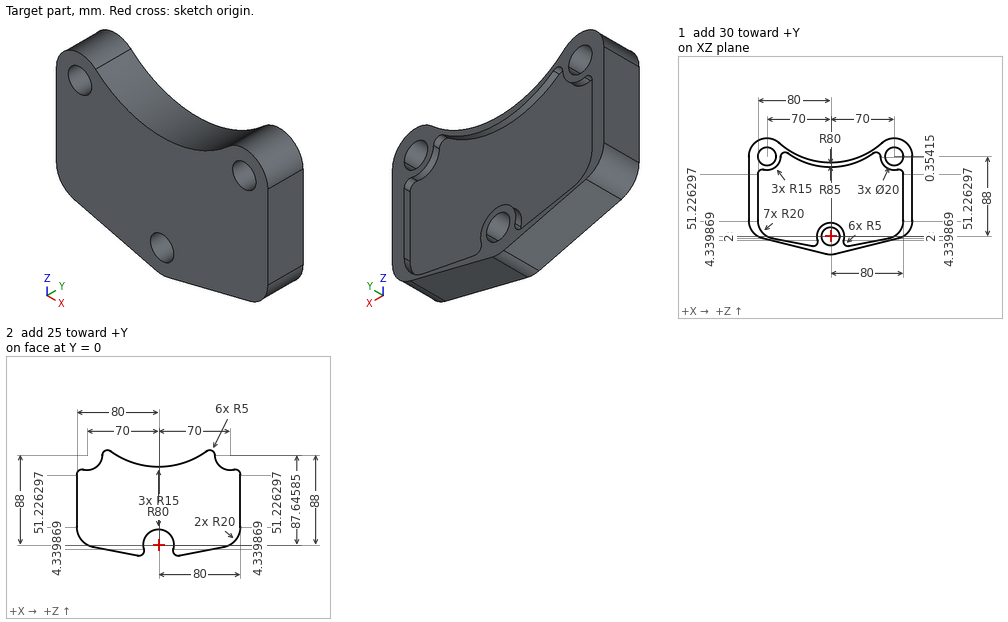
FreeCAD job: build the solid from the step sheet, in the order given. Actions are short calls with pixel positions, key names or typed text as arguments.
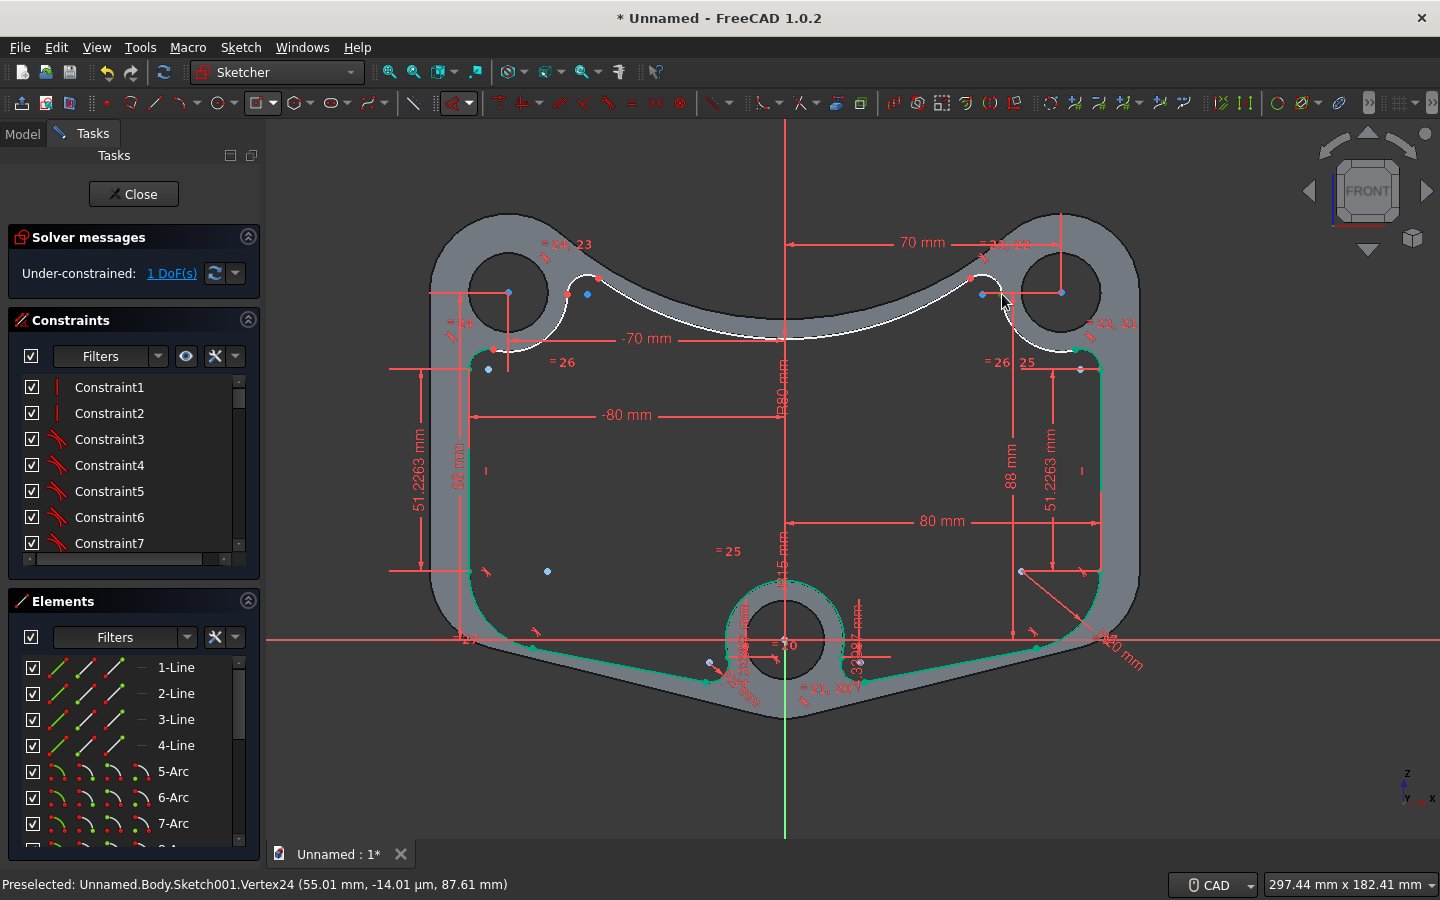
key(i)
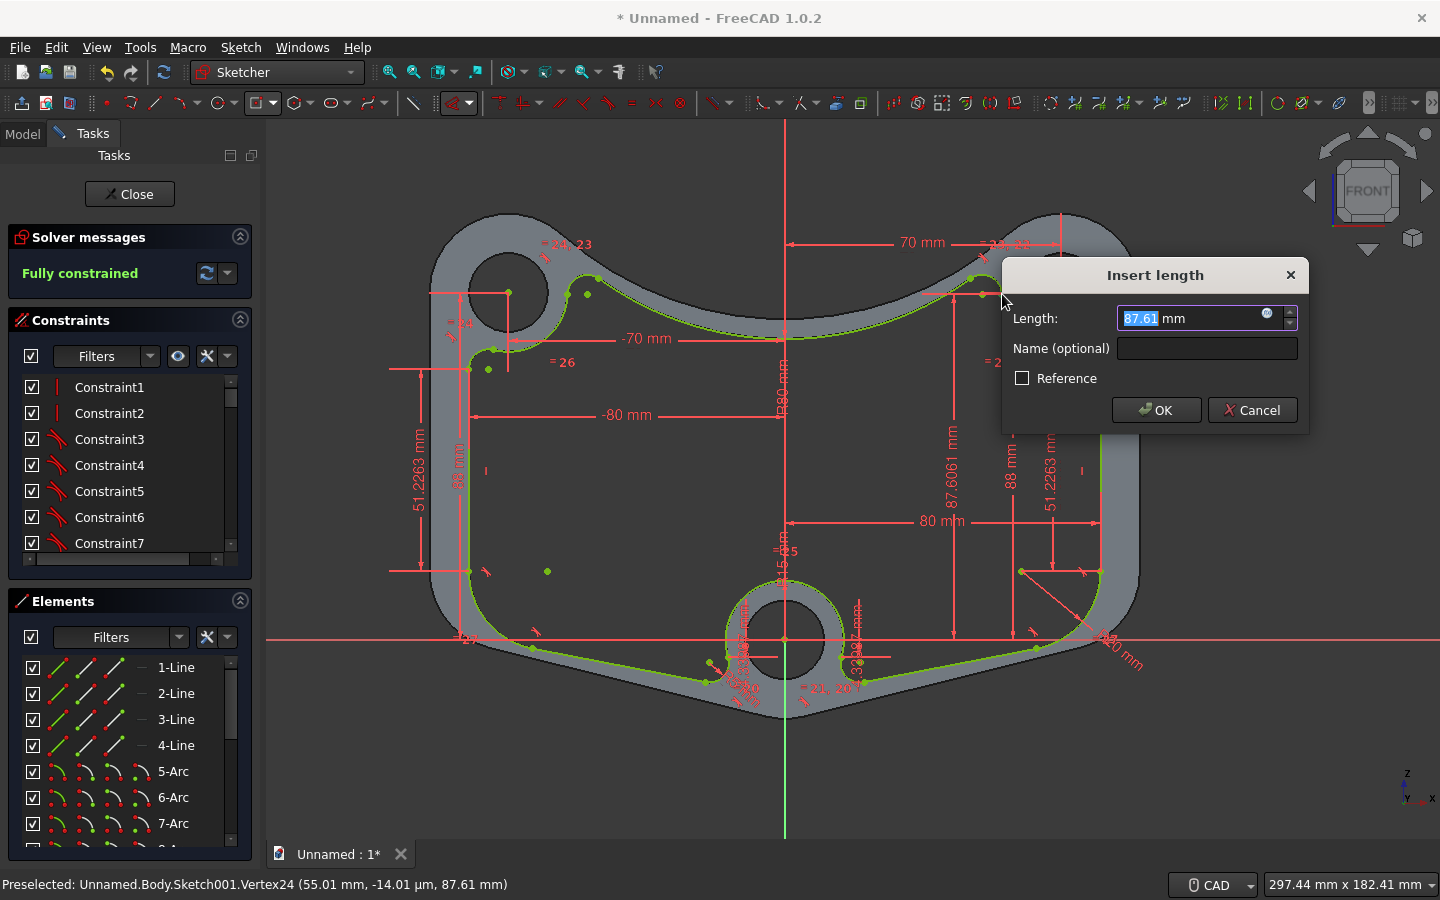
text(87.64585)
key(Return)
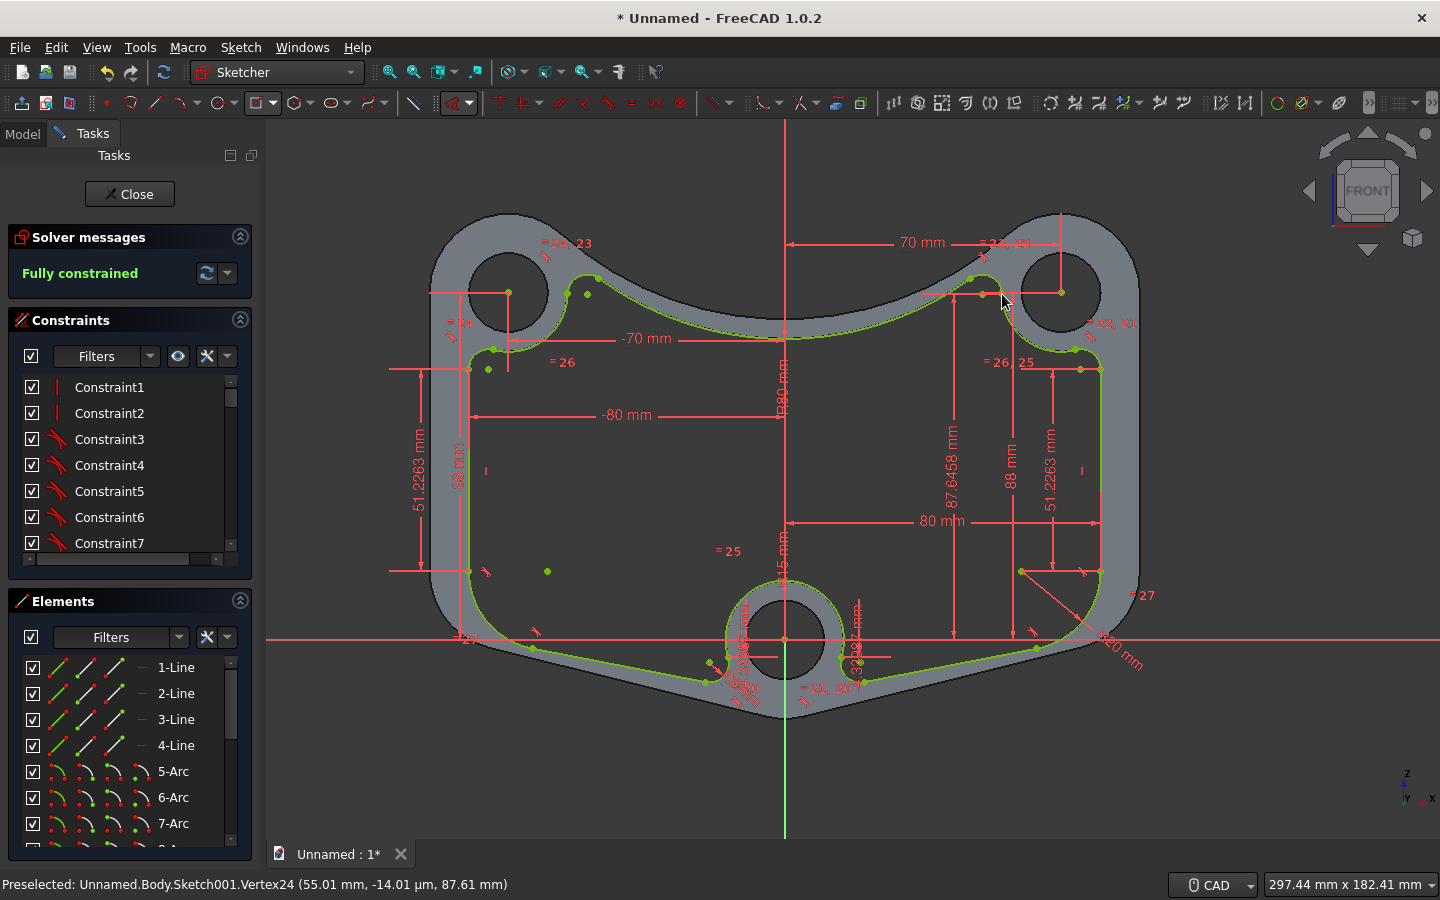
click(130, 194)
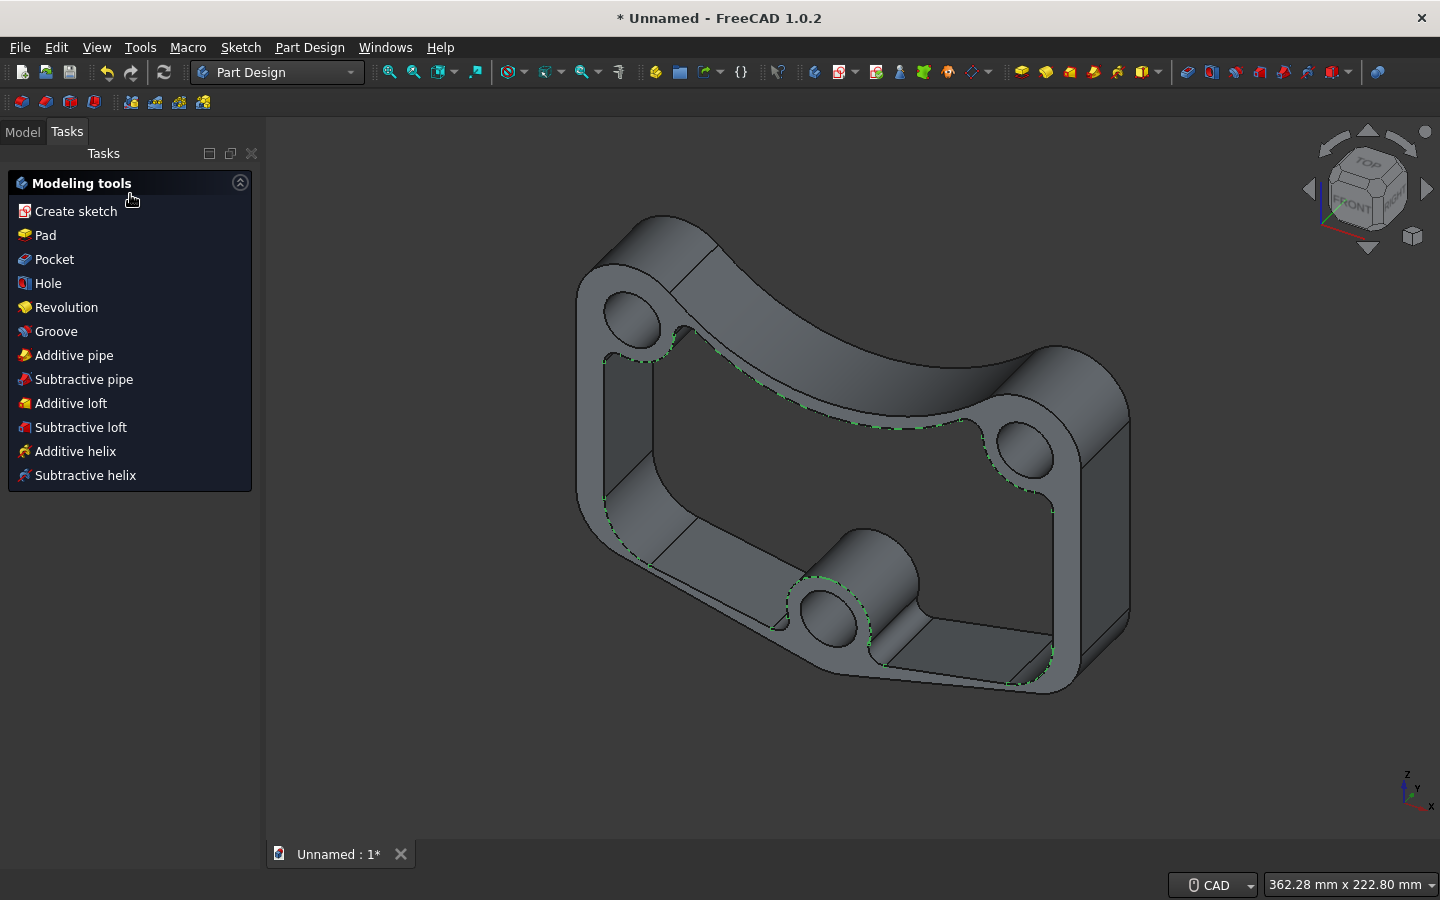
click(1022, 72)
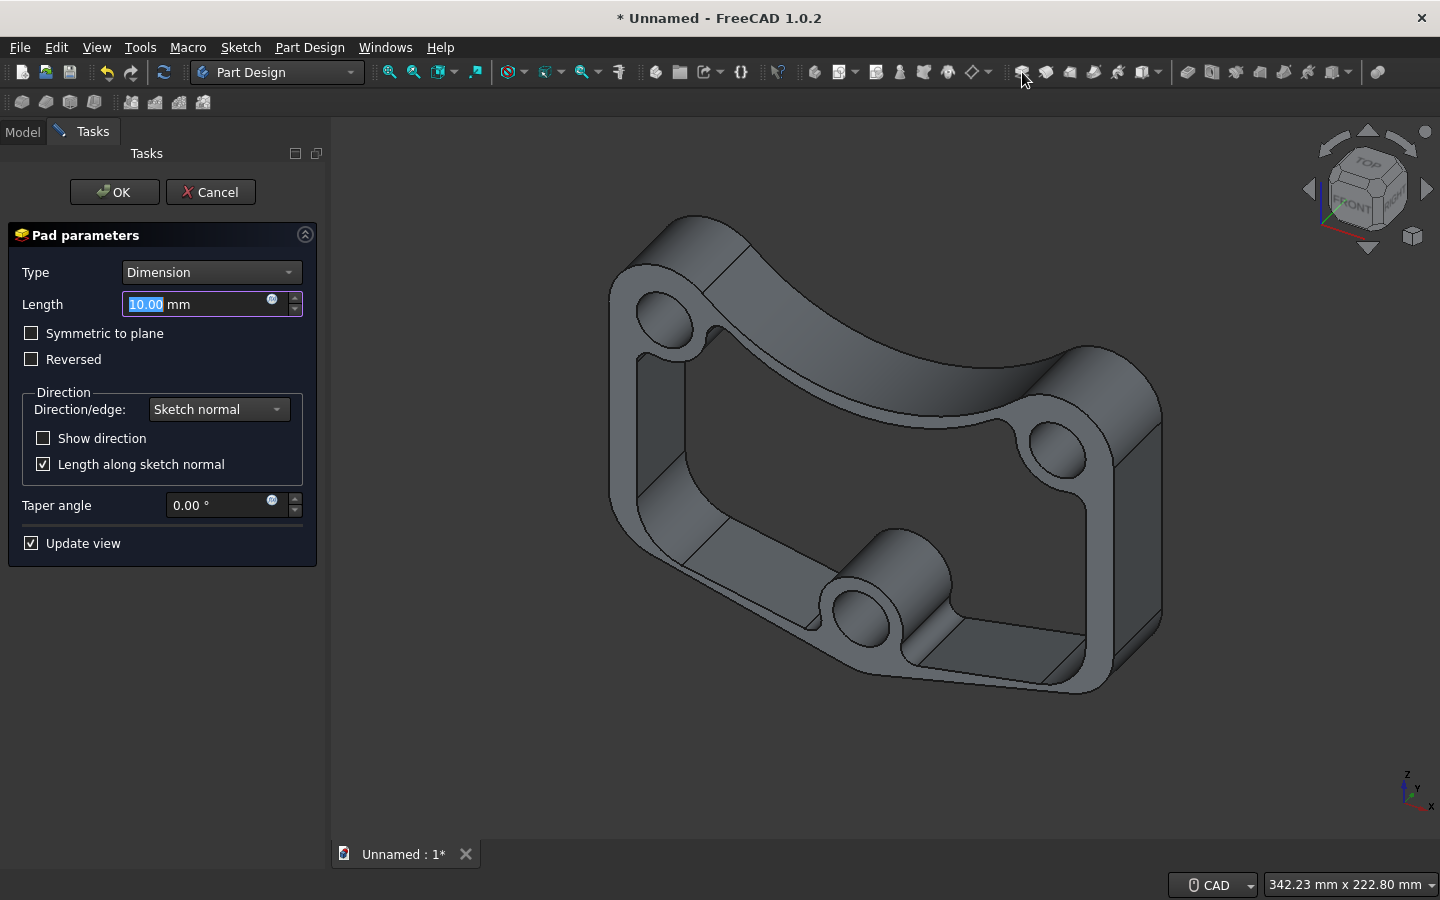
text(25)
key(Tab)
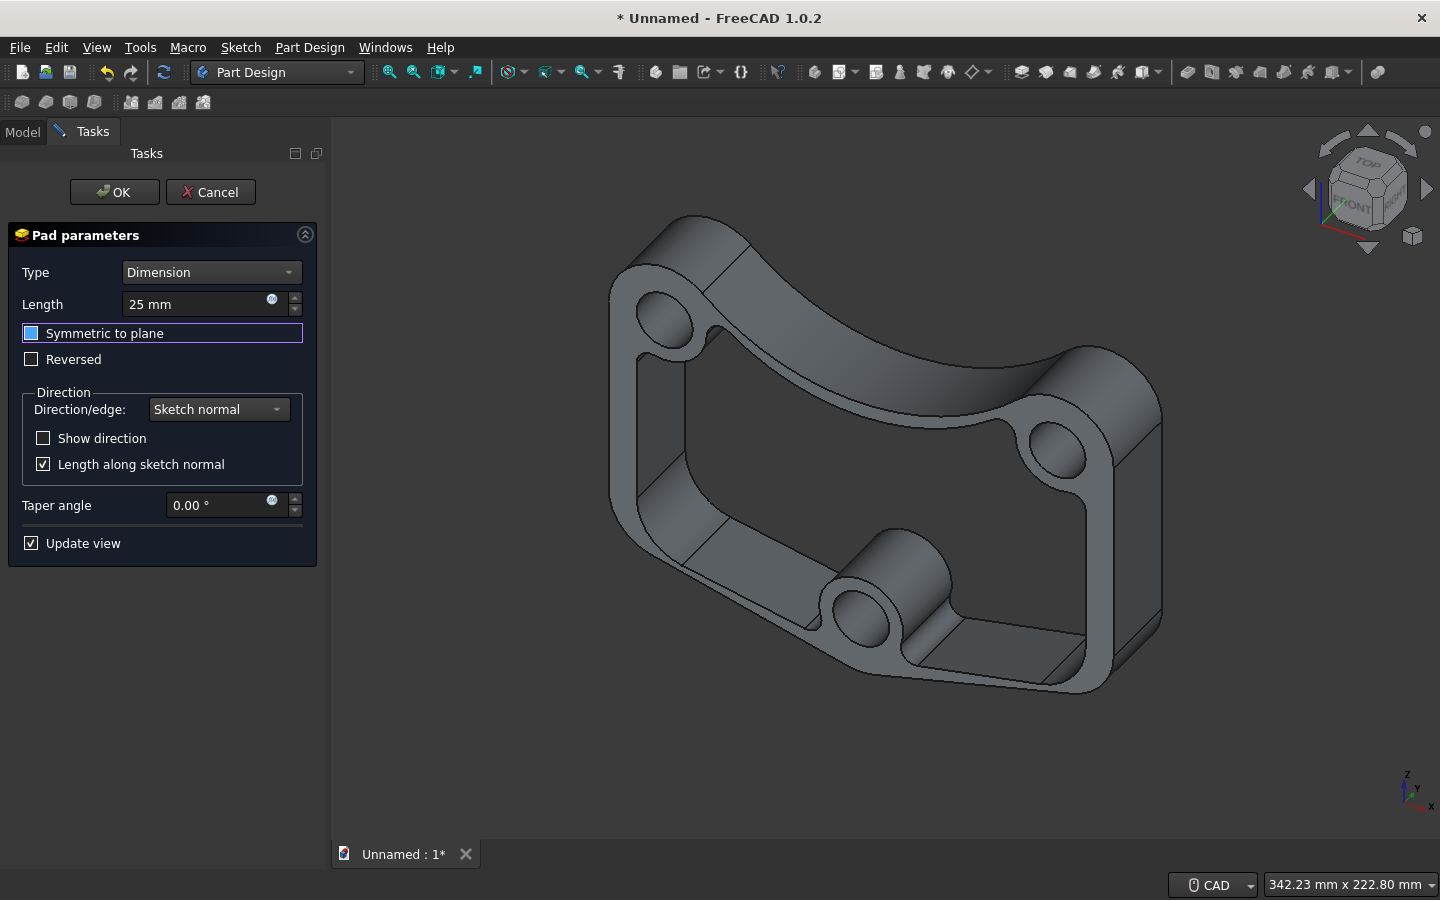
click(30, 359)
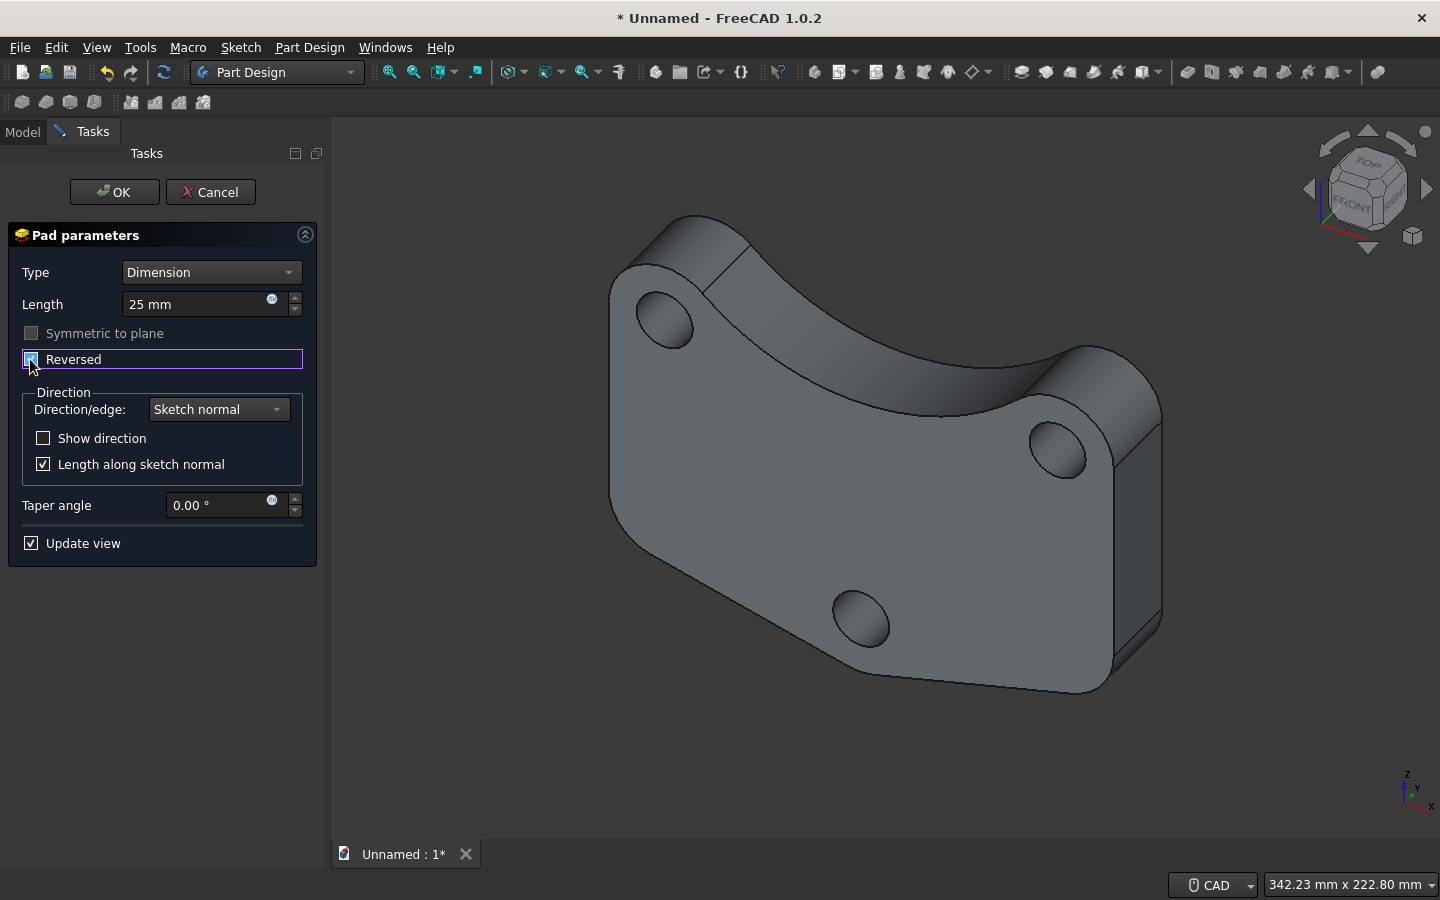
click(115, 192)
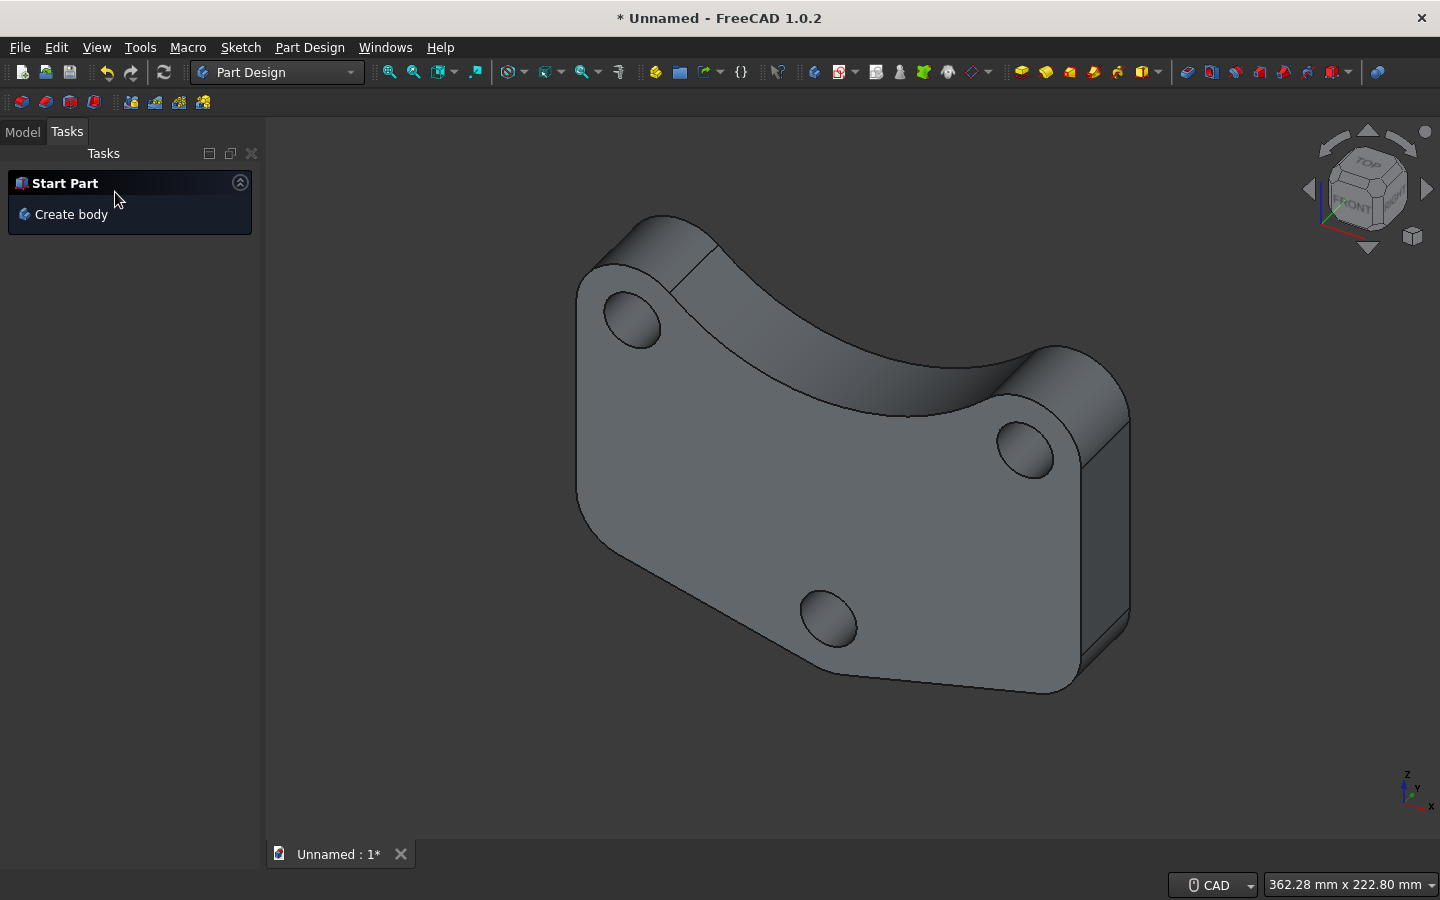
key(0)